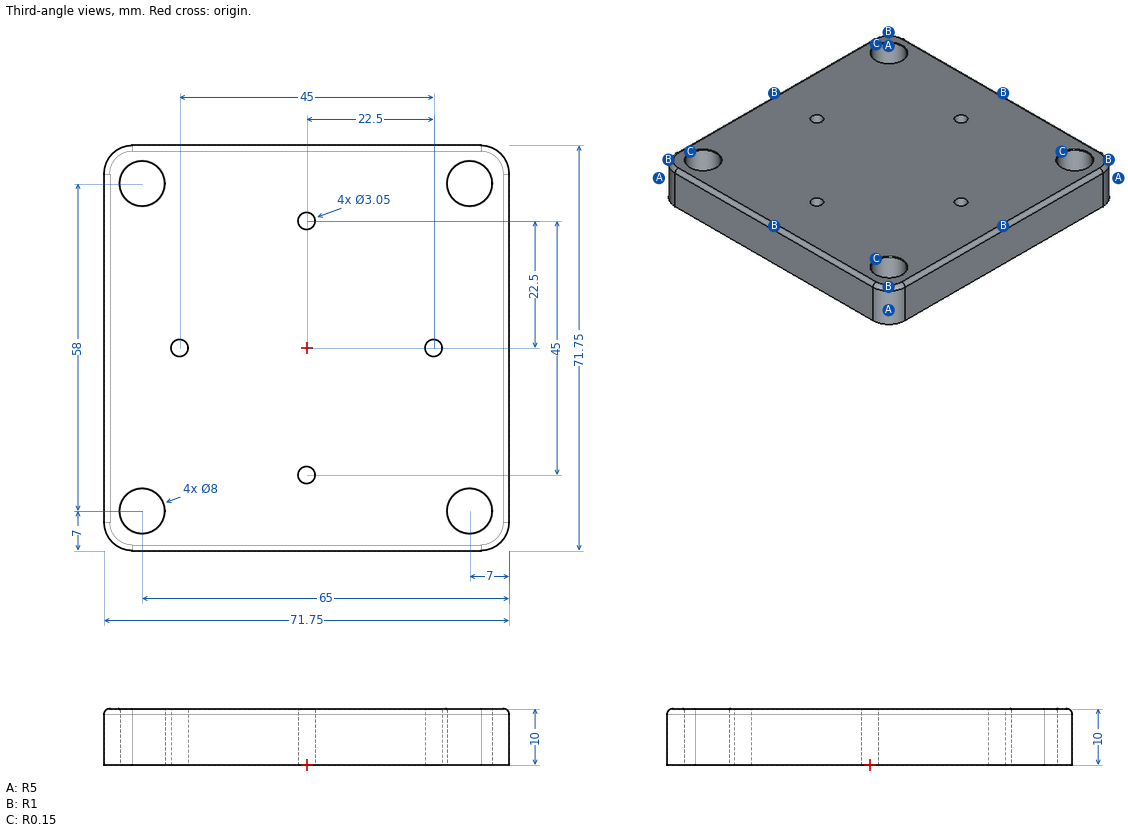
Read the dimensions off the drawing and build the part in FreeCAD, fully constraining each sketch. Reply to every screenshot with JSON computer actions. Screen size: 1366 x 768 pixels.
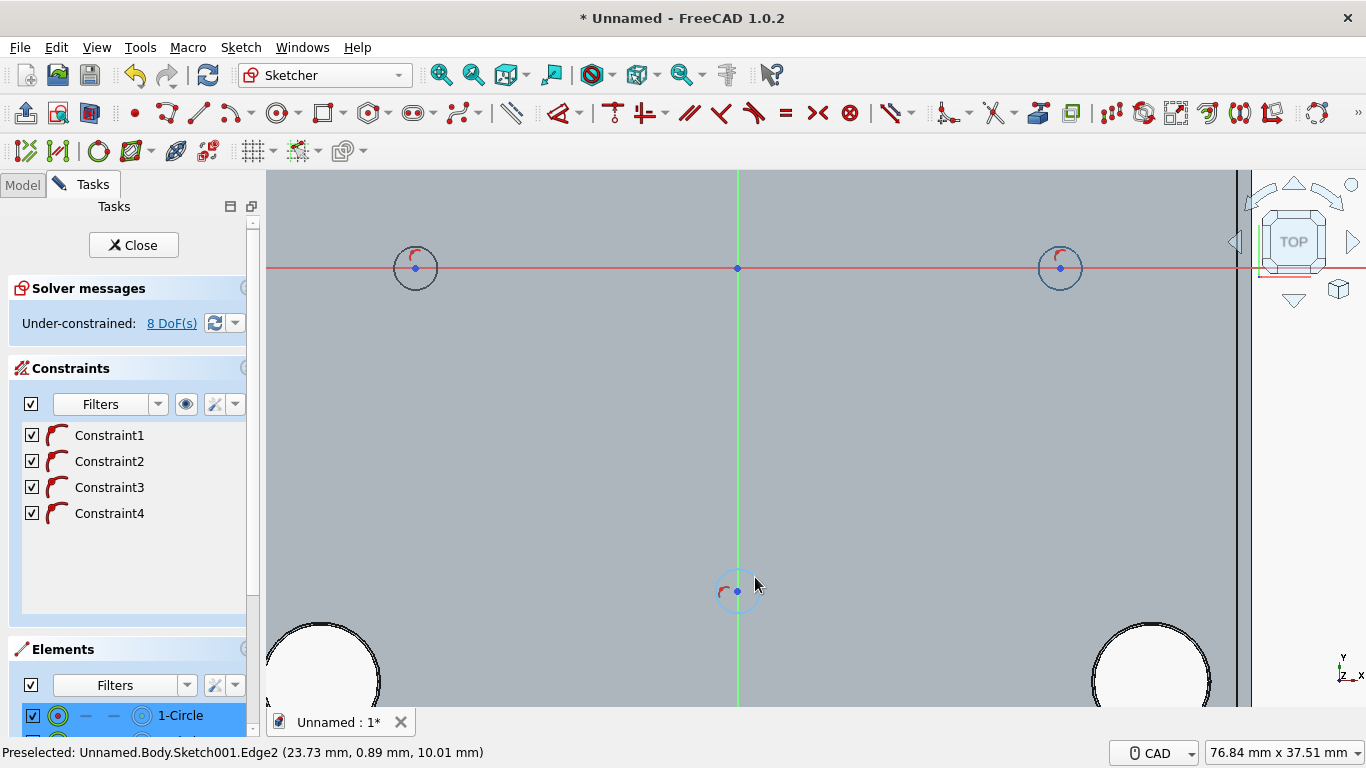
{"action": "left_click", "coordinate": [753, 576]}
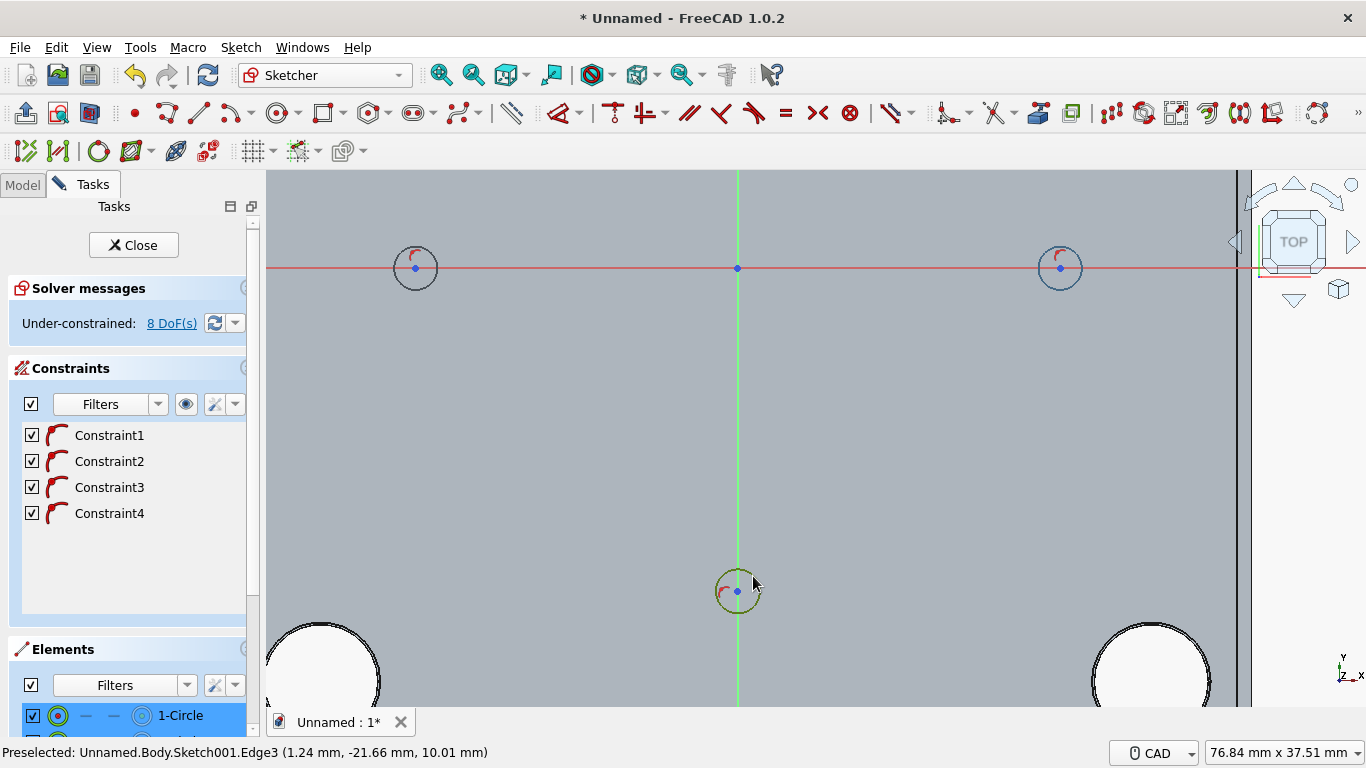
{"action": "left_click", "coordinate": [431, 253]}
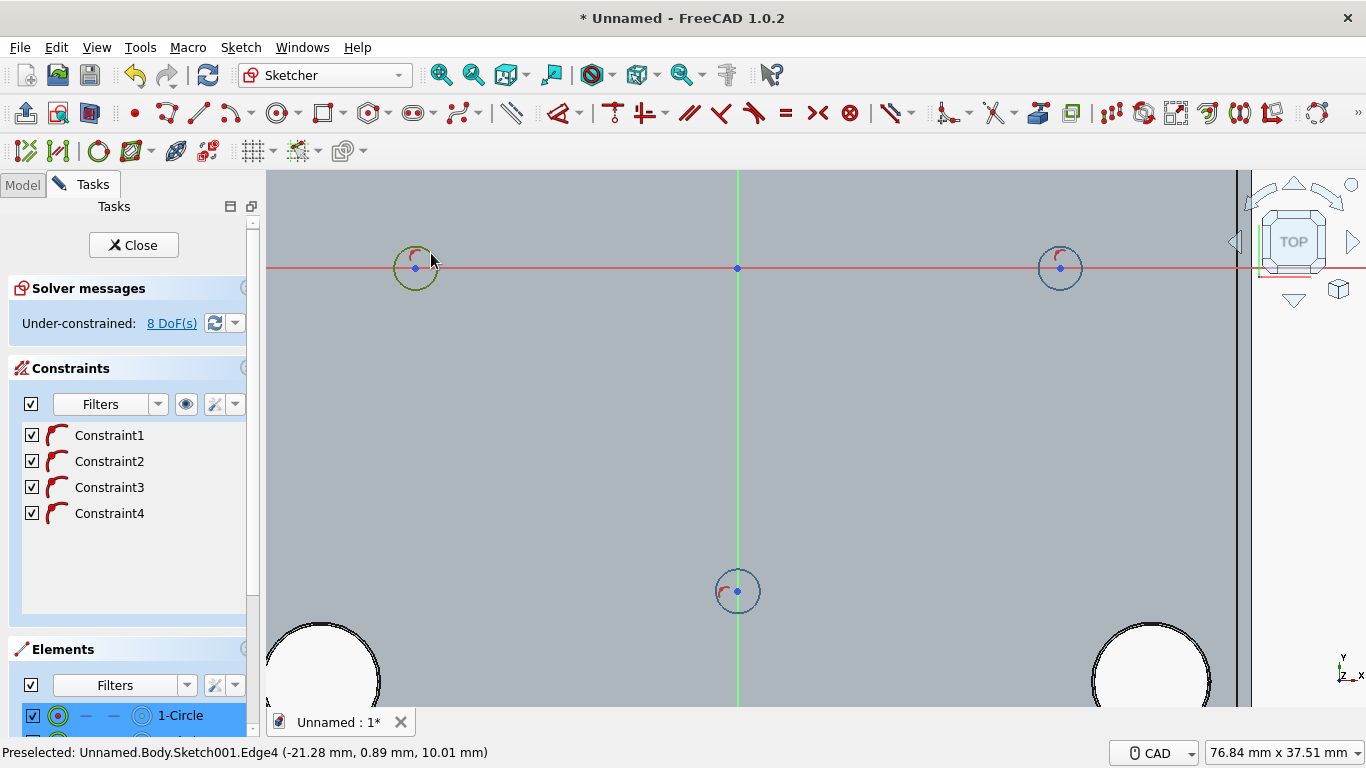
{"action": "left_click", "coordinate": [786, 114]}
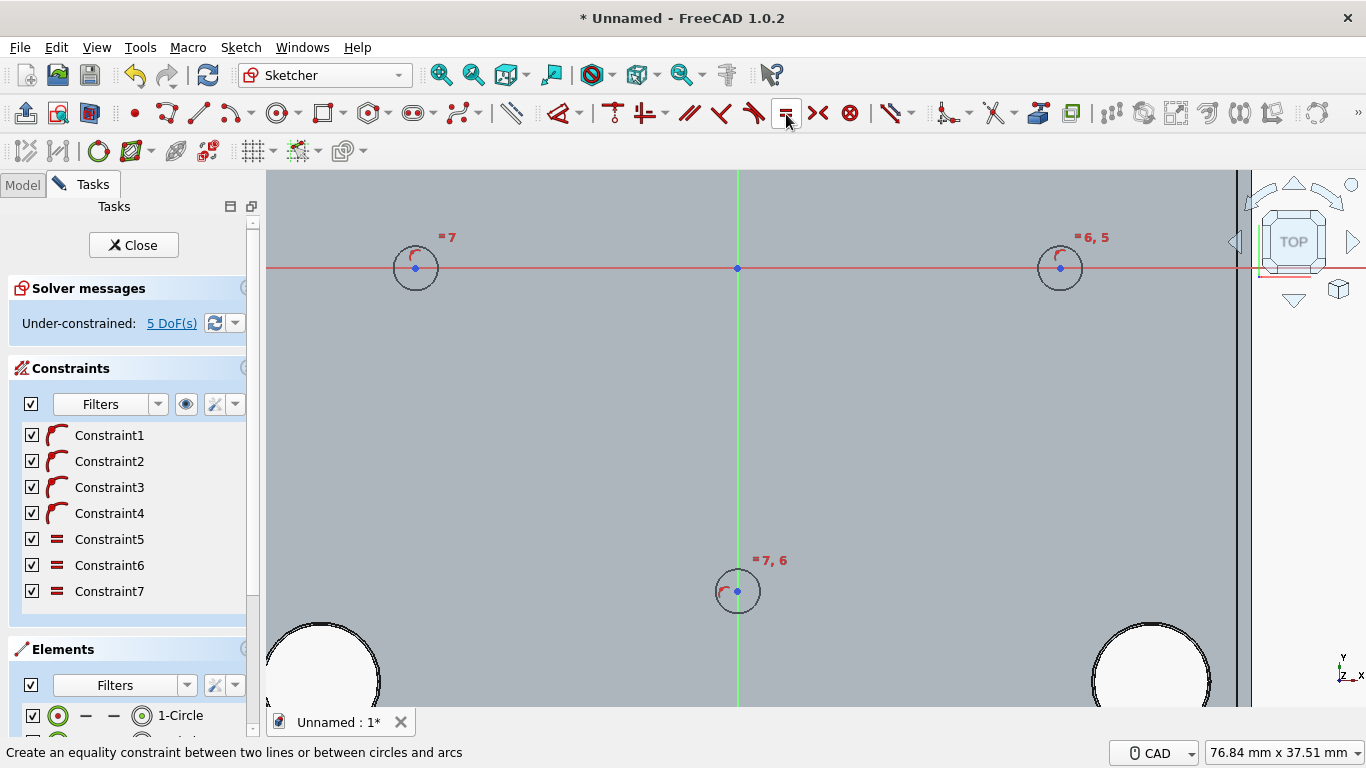
{"action": "left_click", "coordinate": [558, 114]}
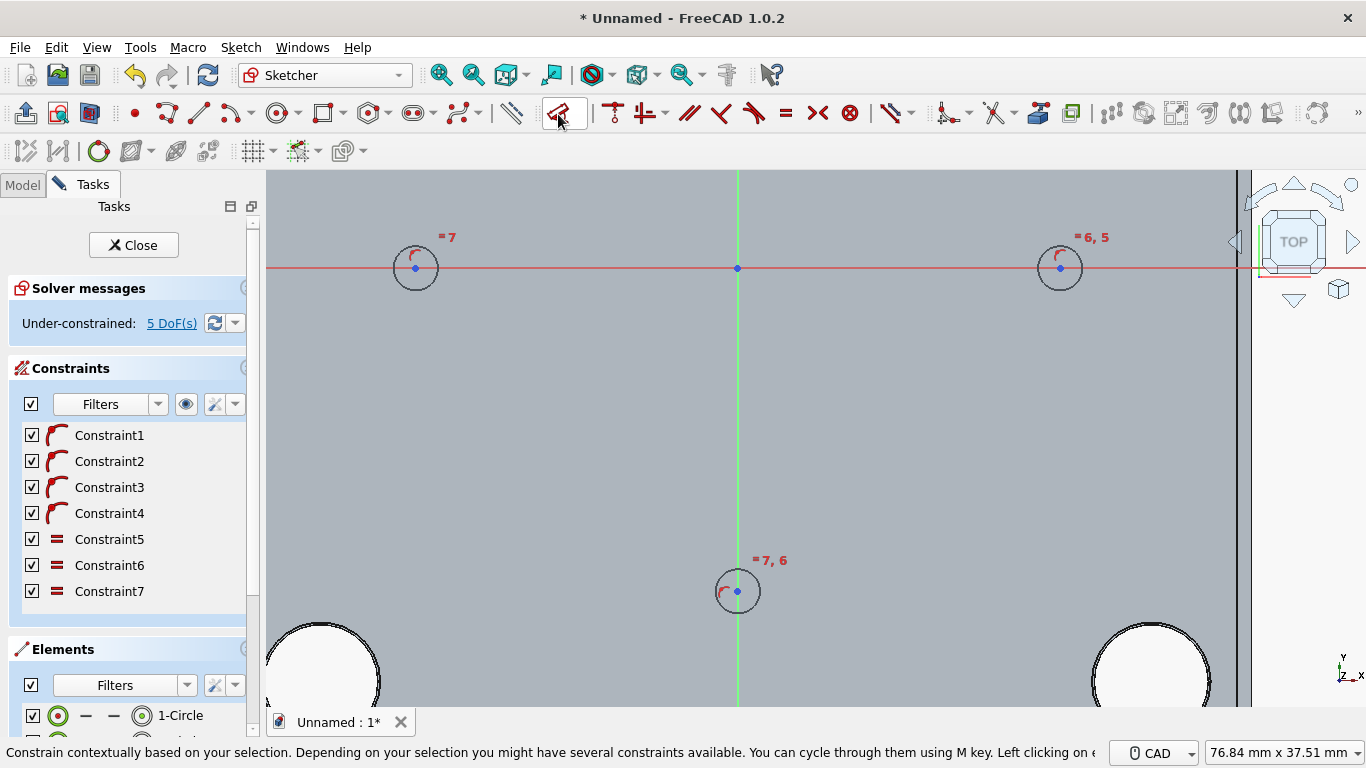
{"action": "scroll", "coordinate": [755, 577], "scroll_direction": "down", "scroll_amount": 4}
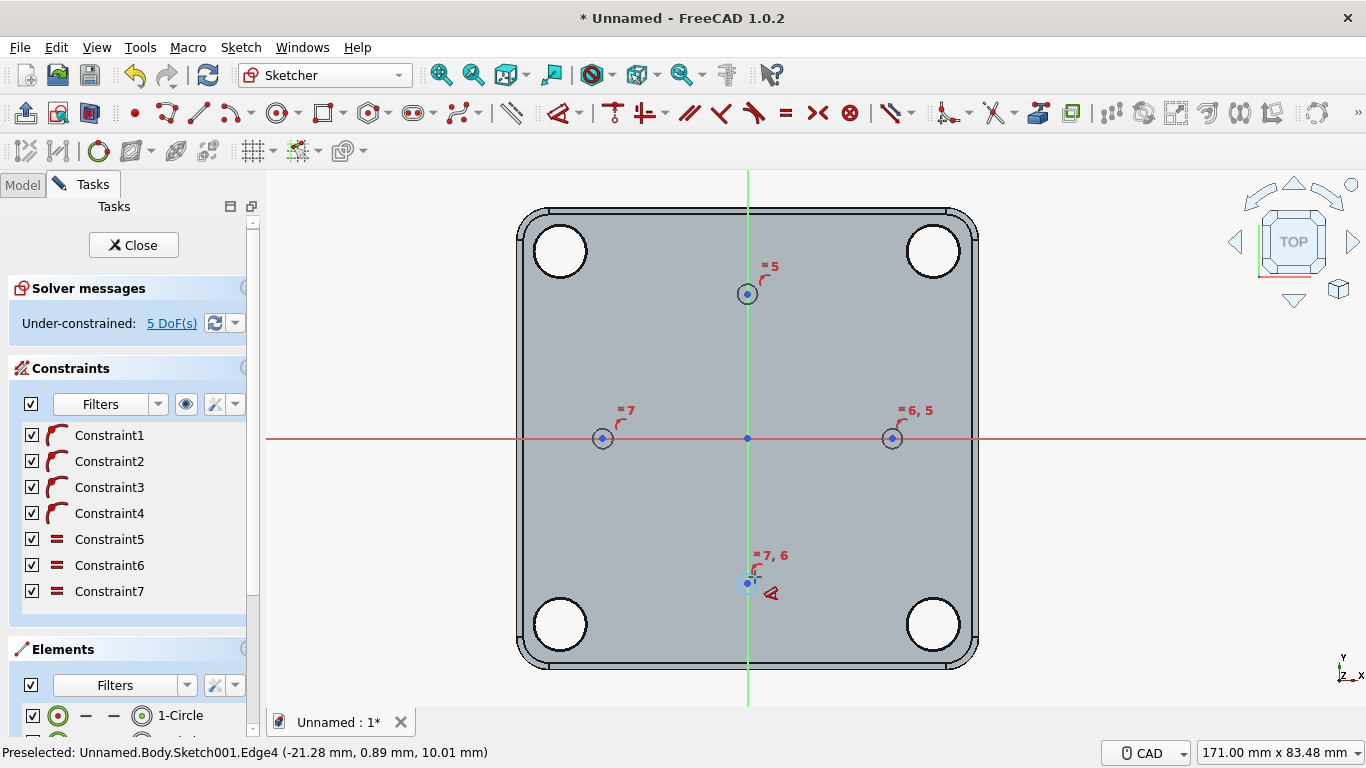
{"action": "scroll", "coordinate": [755, 287], "scroll_direction": "up", "scroll_amount": 4}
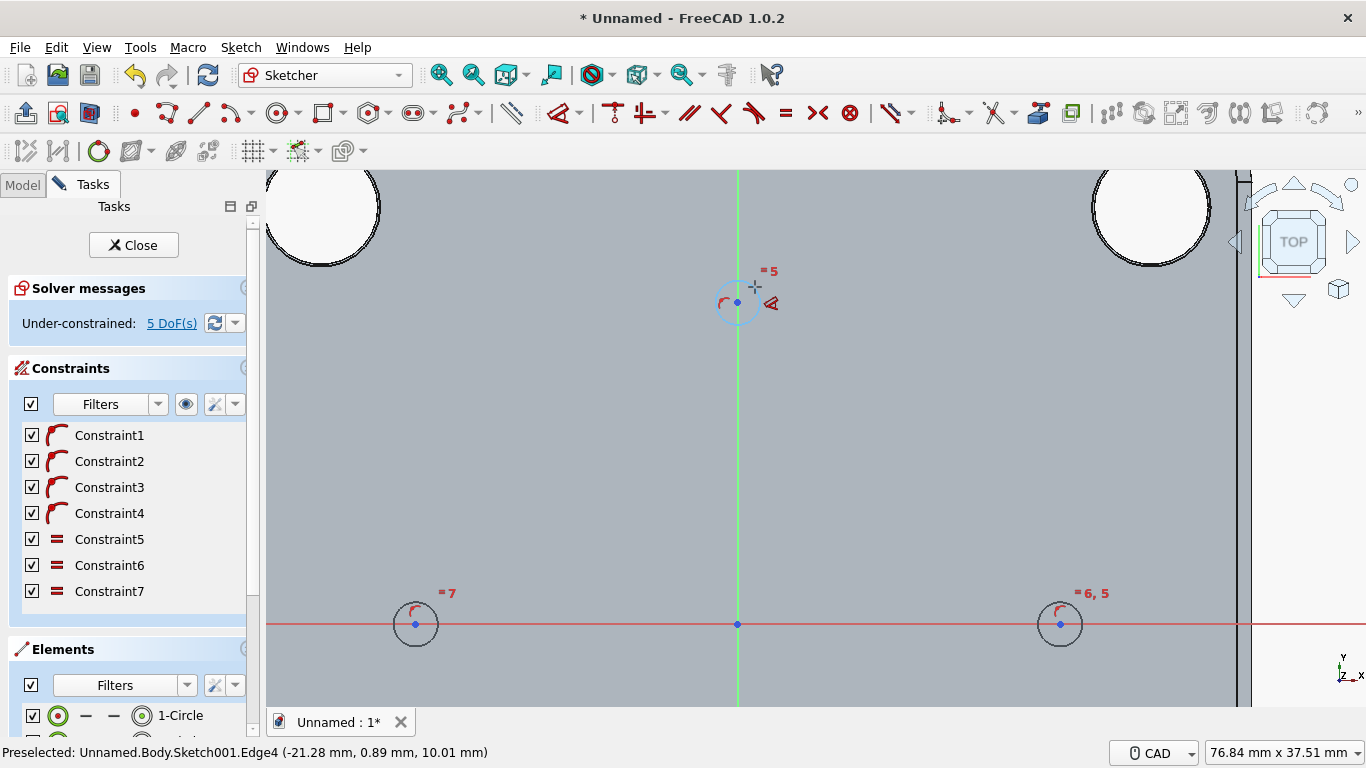
{"action": "left_click", "coordinate": [753, 287]}
{"action": "left_click", "coordinate": [775, 264]}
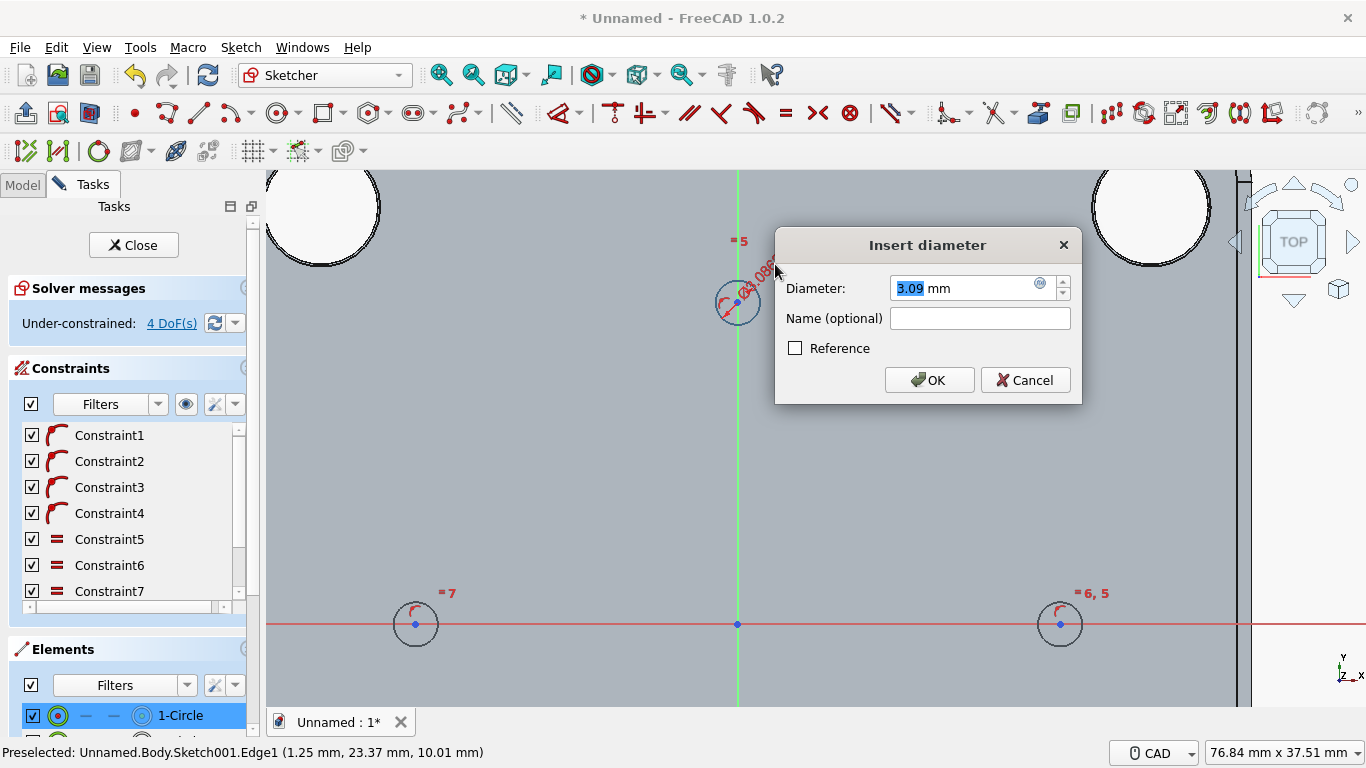
{"action": "type", "text": "3.05"}
{"action": "key", "text": "Return"}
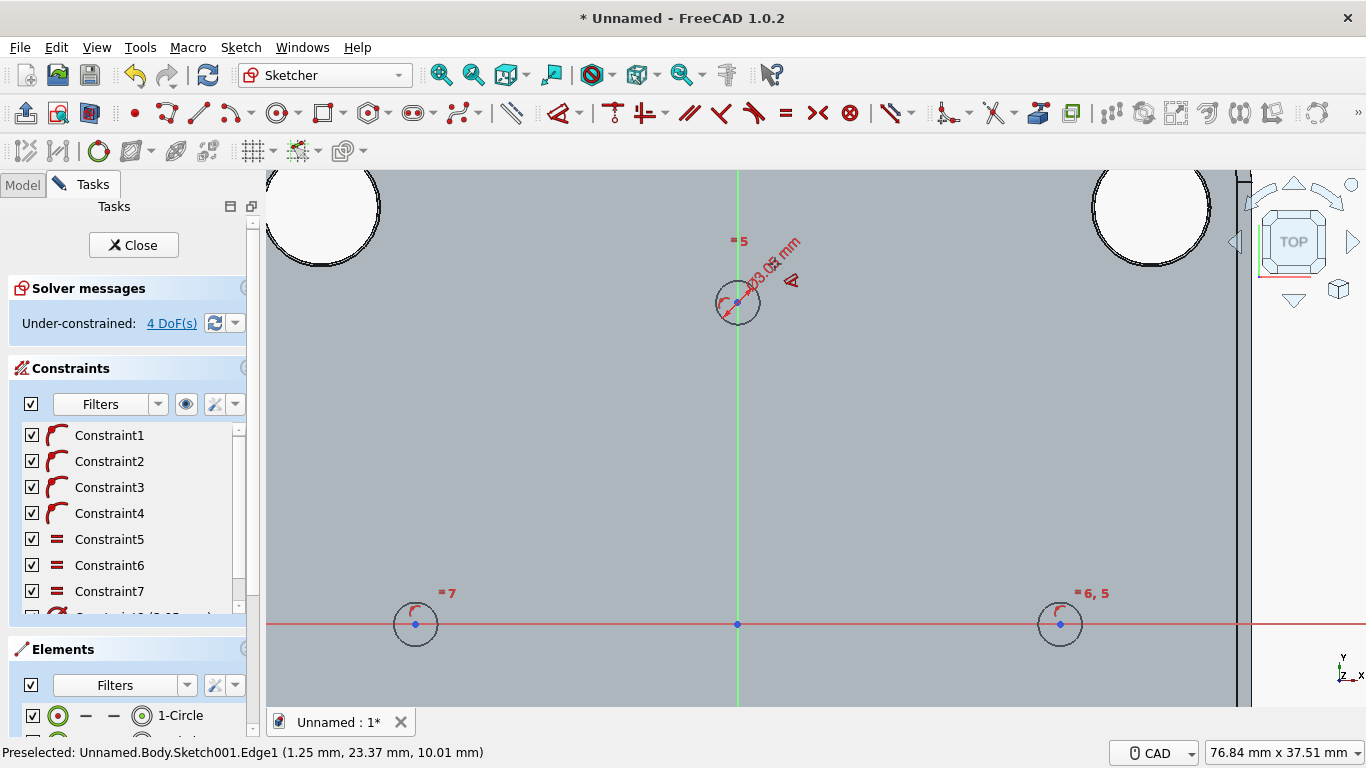
{"action": "left_click", "coordinate": [738, 303]}